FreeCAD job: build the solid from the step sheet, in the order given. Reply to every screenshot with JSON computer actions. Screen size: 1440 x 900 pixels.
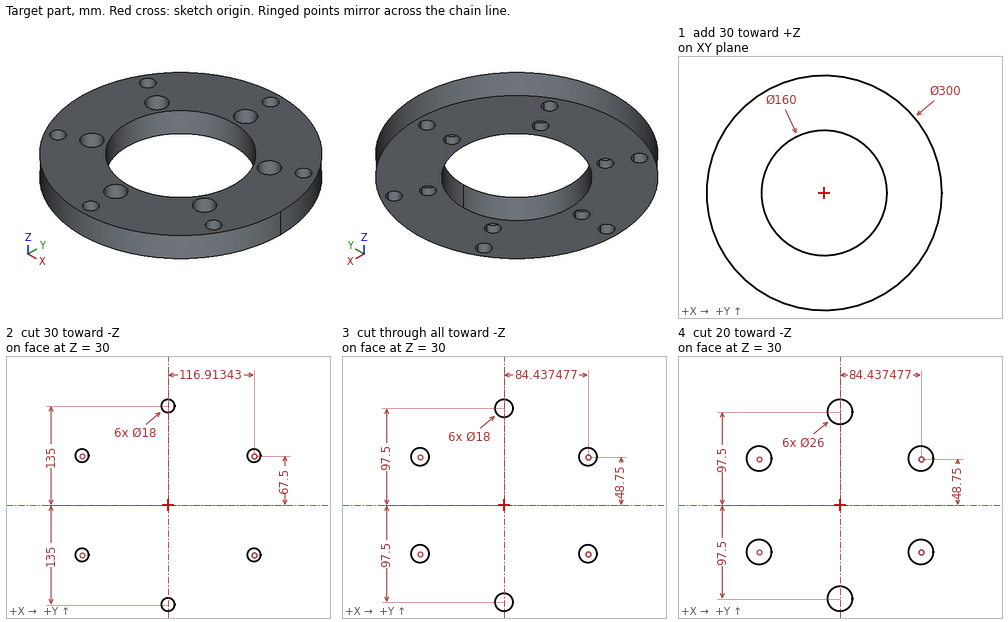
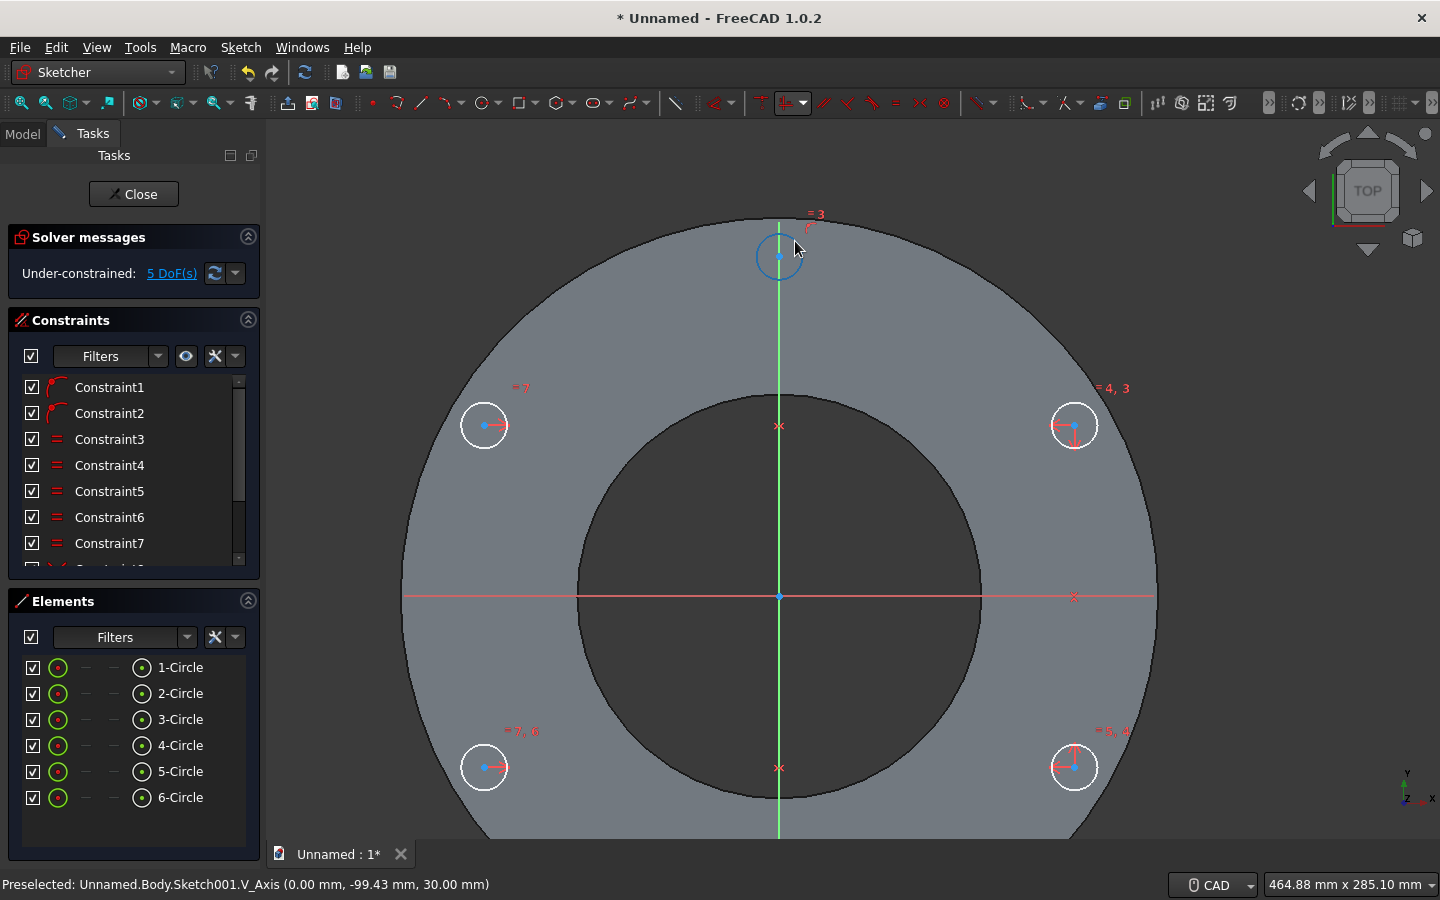
{"action": "left_click", "coordinate": [795, 241]}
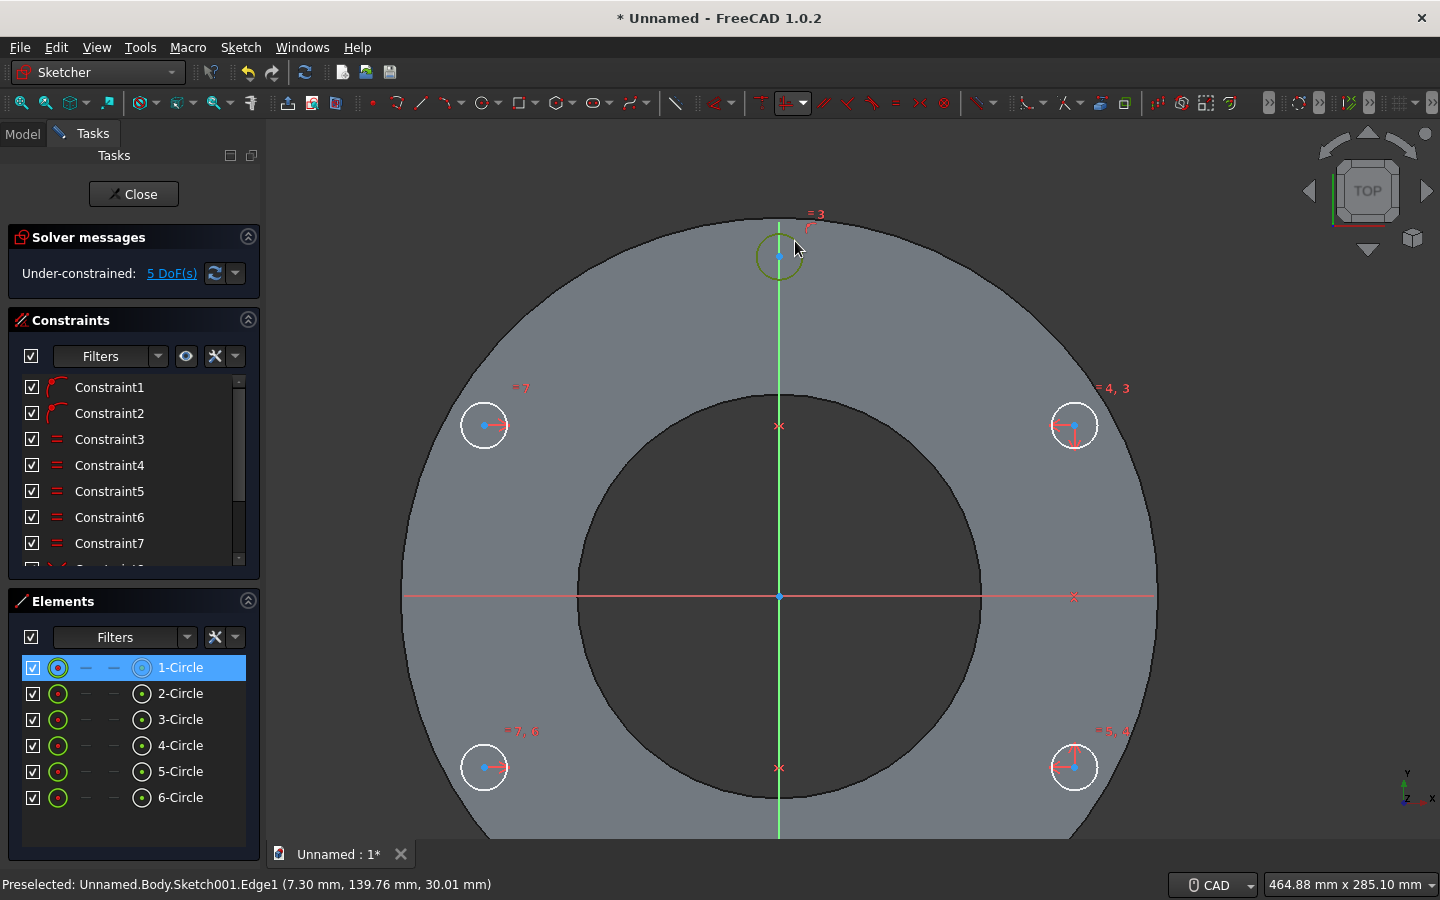
{"action": "key", "text": "k o"}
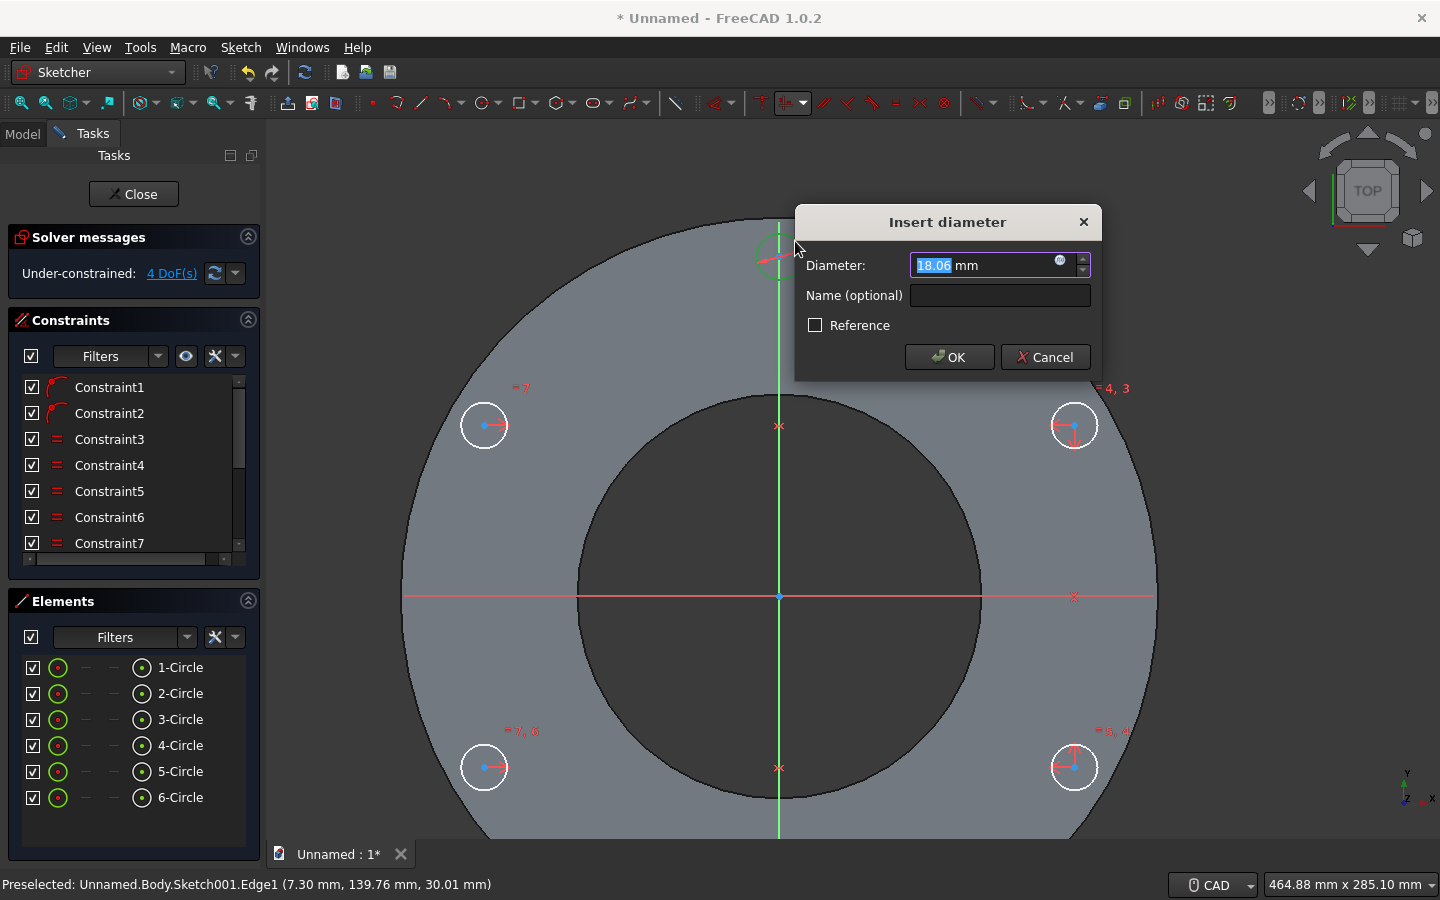
{"action": "type", "text": "18"}
{"action": "key", "text": "Return"}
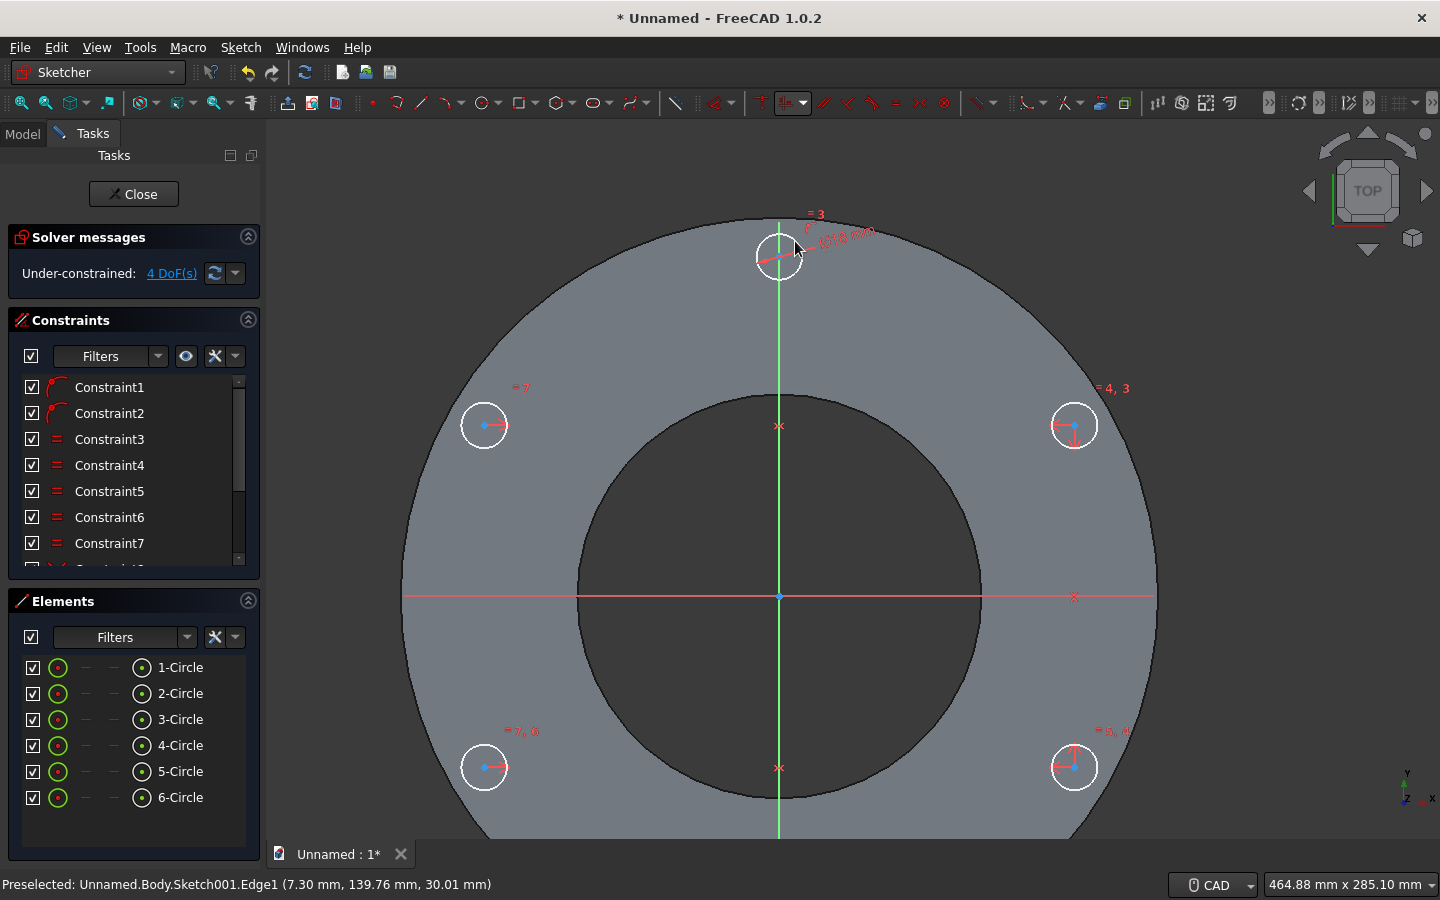
{"action": "left_click", "coordinate": [779, 257]}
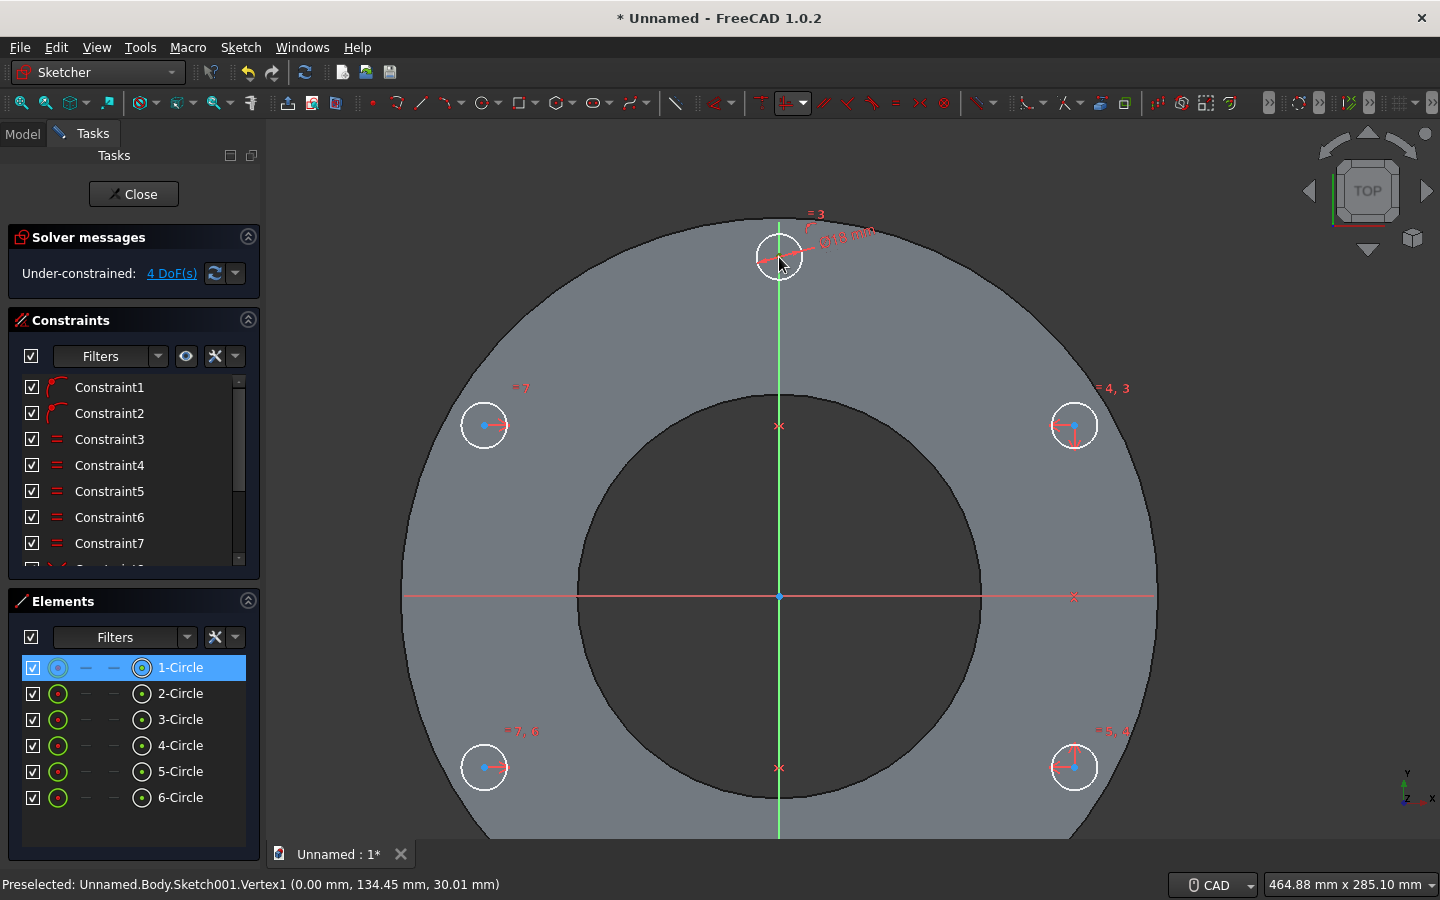
{"action": "key", "text": "i"}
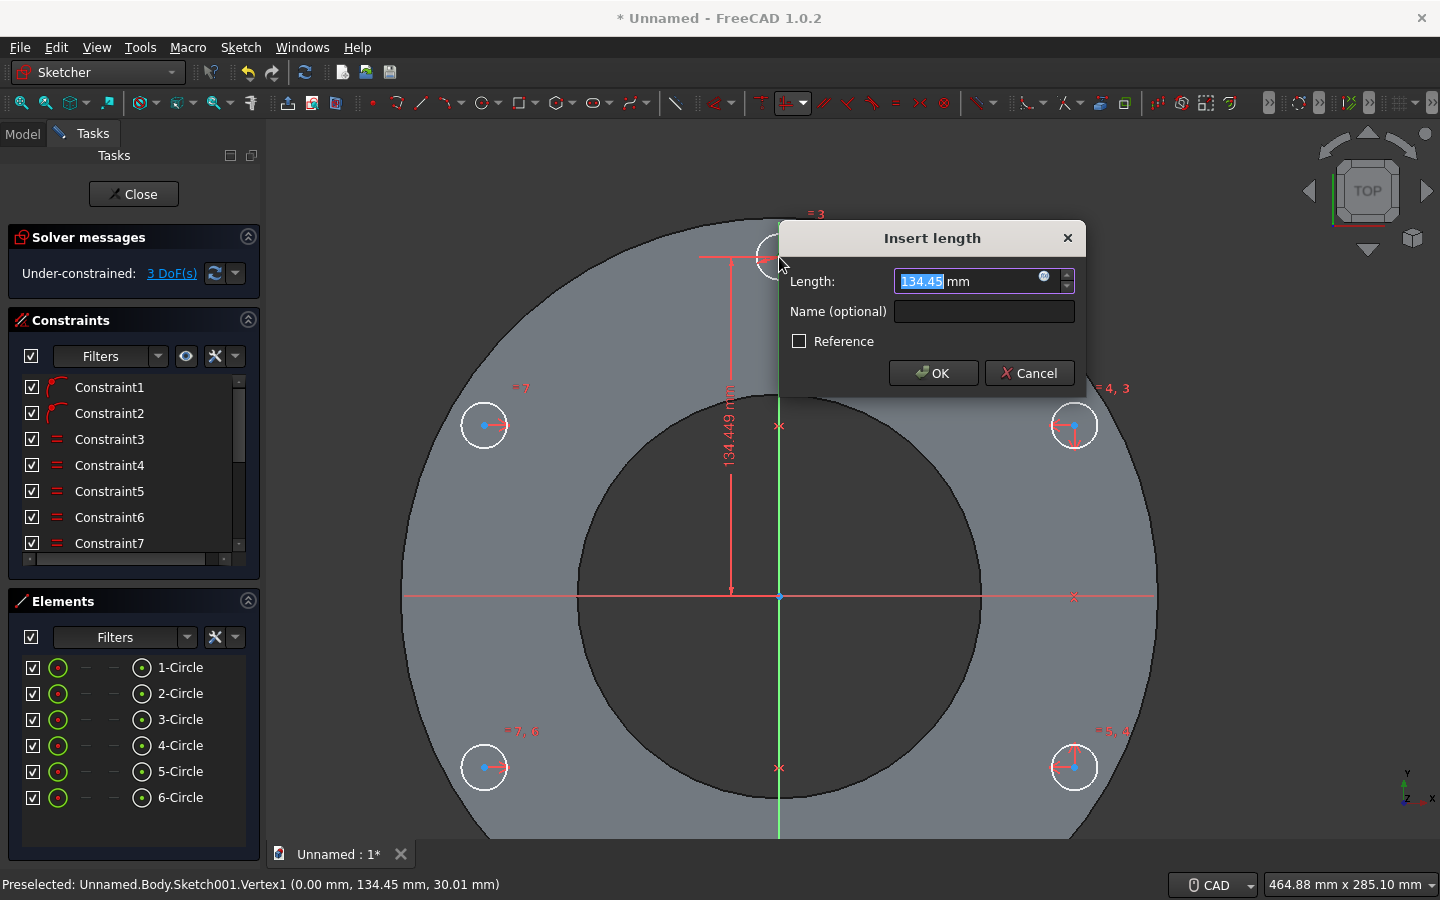
{"action": "type", "text": "135"}
{"action": "key", "text": "Return"}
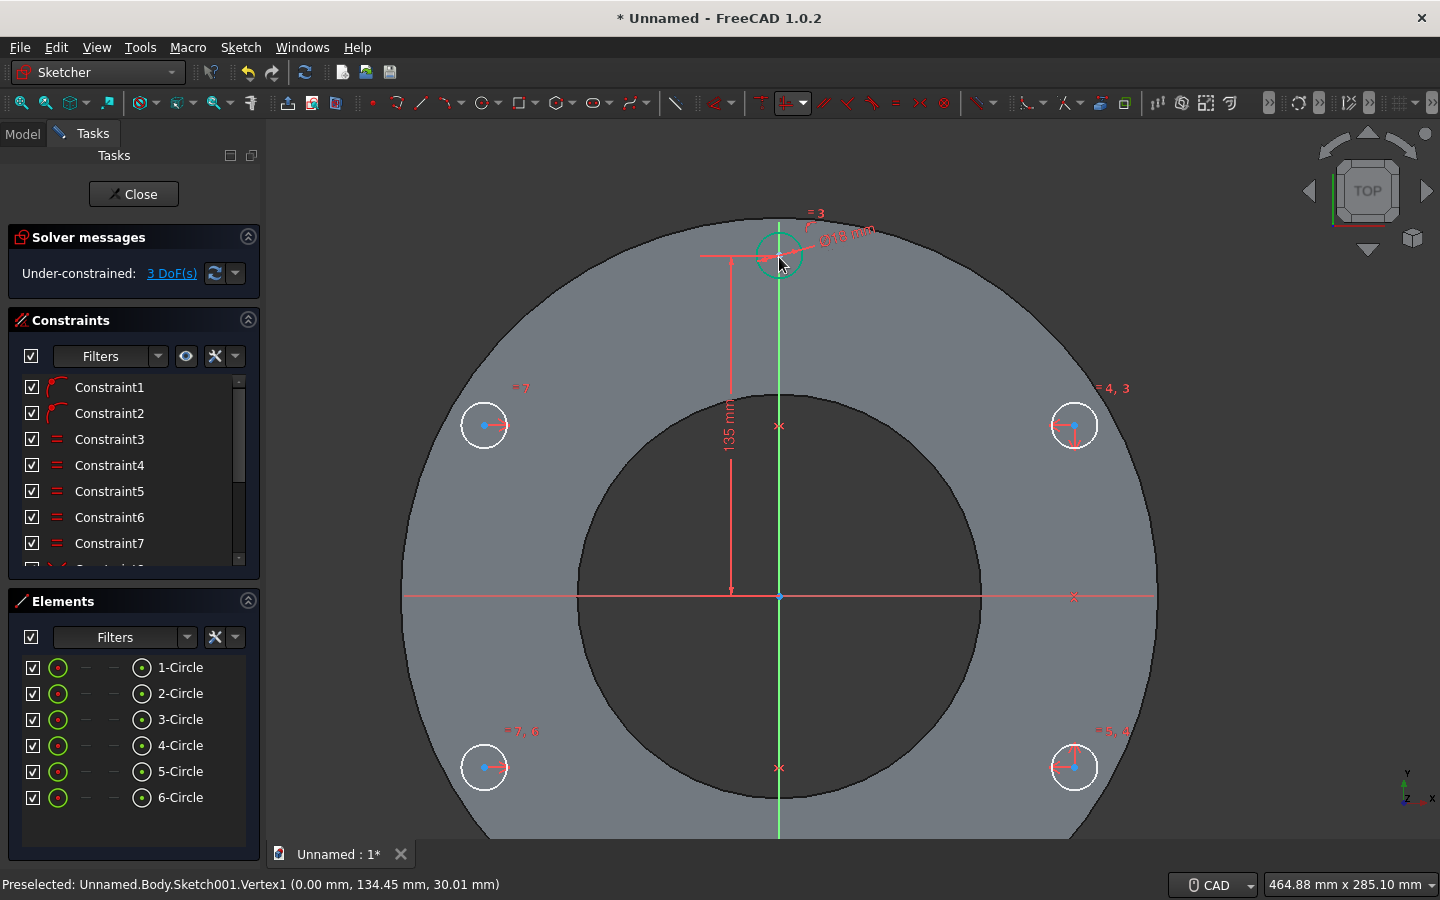
{"action": "scroll", "coordinate": [795, 240], "scroll_direction": "down", "scroll_amount": 2}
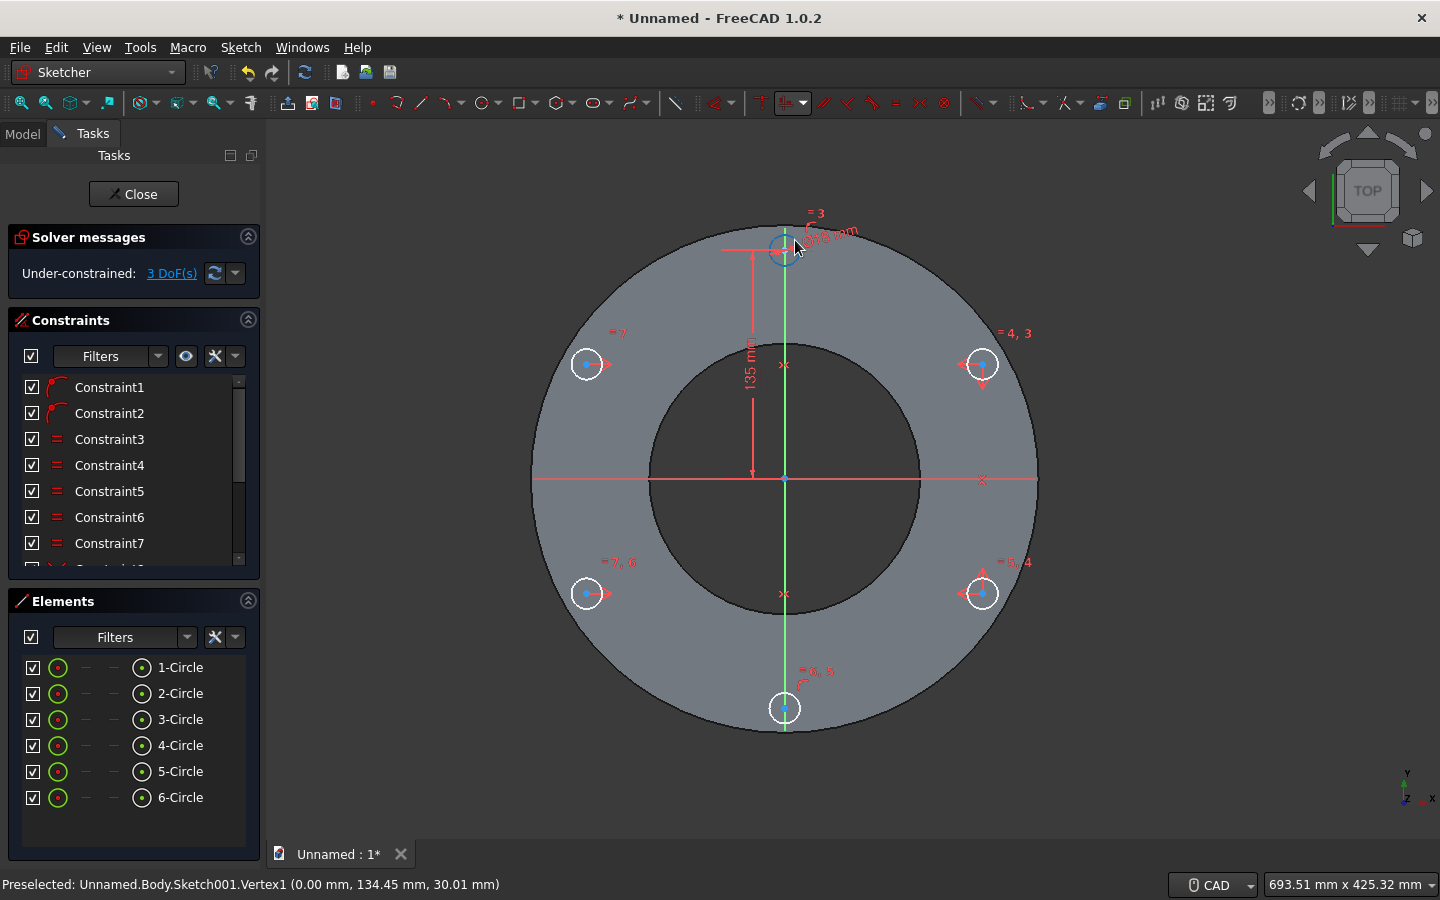
{"action": "left_click", "coordinate": [785, 708]}